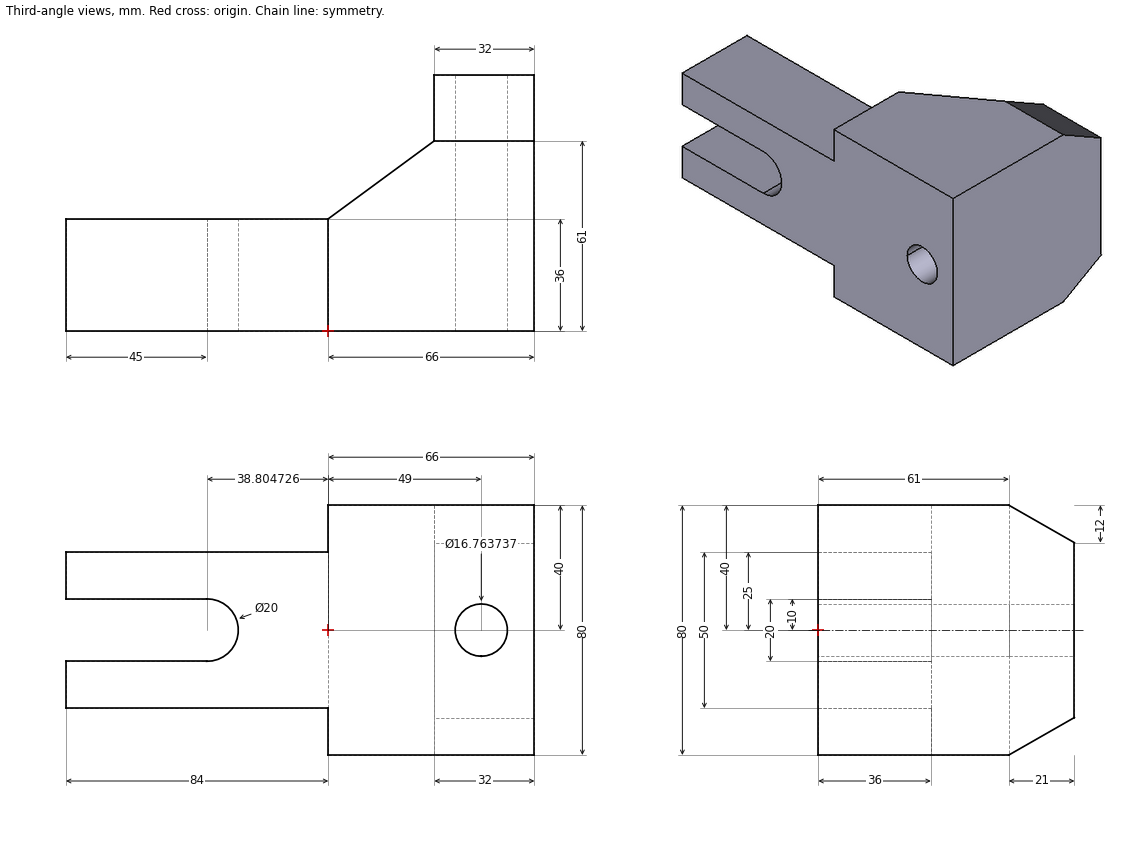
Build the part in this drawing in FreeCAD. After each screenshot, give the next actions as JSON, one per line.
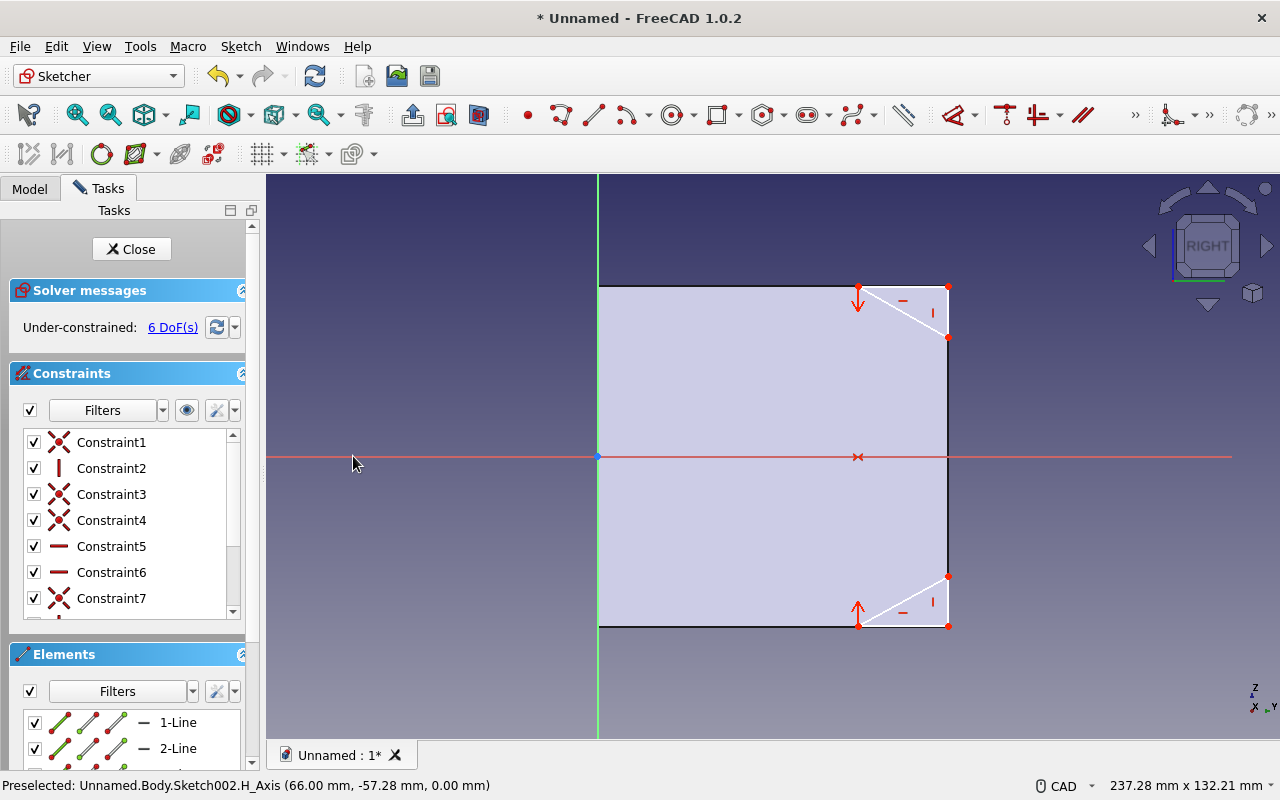
{"action": "left_click", "coordinate": [948, 338]}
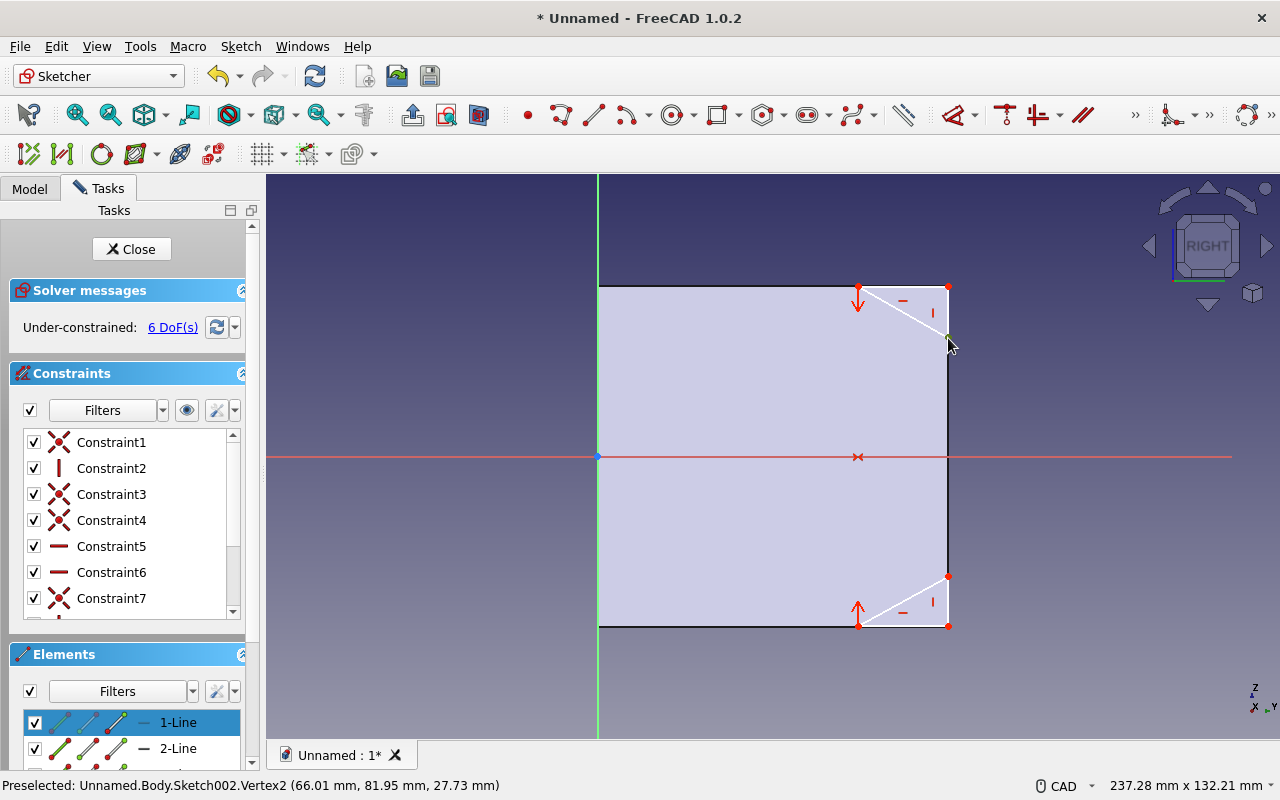
{"action": "left_click", "coordinate": [948, 577]}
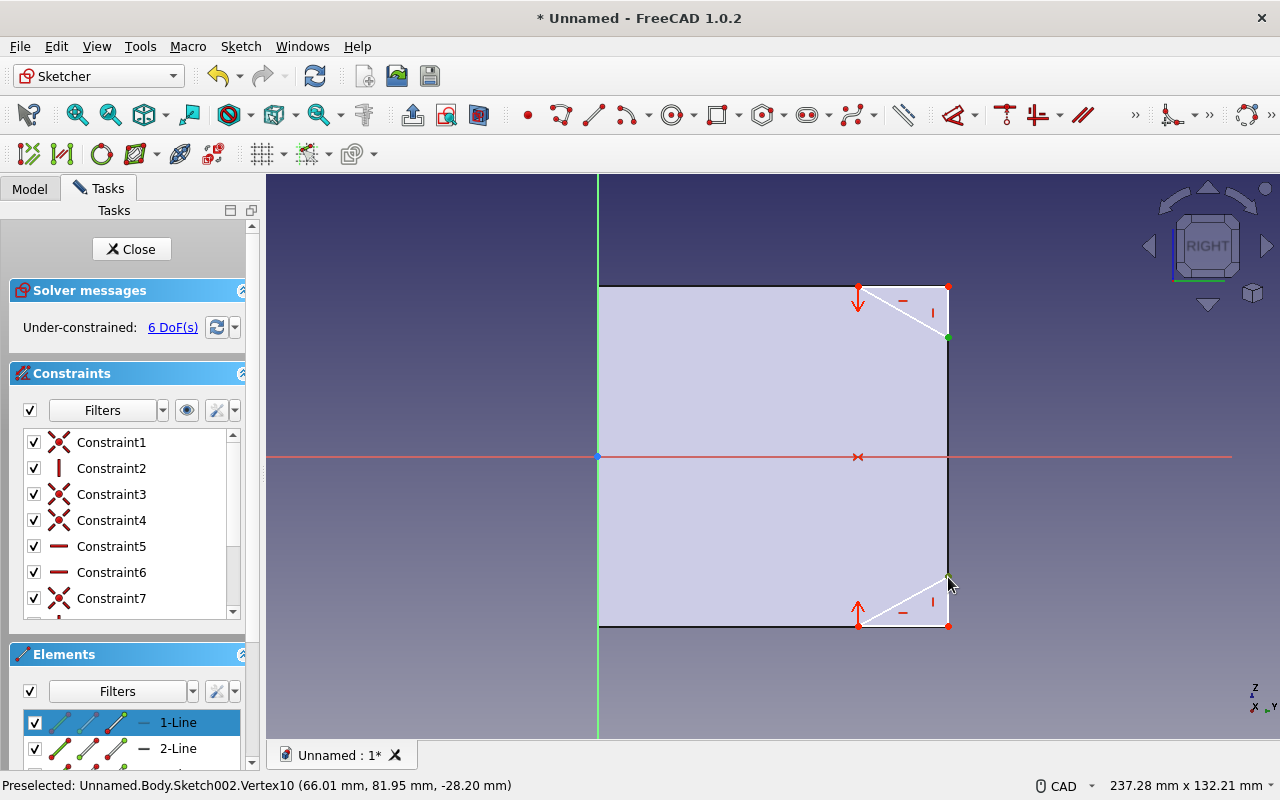
{"action": "left_click", "coordinate": [353, 456]}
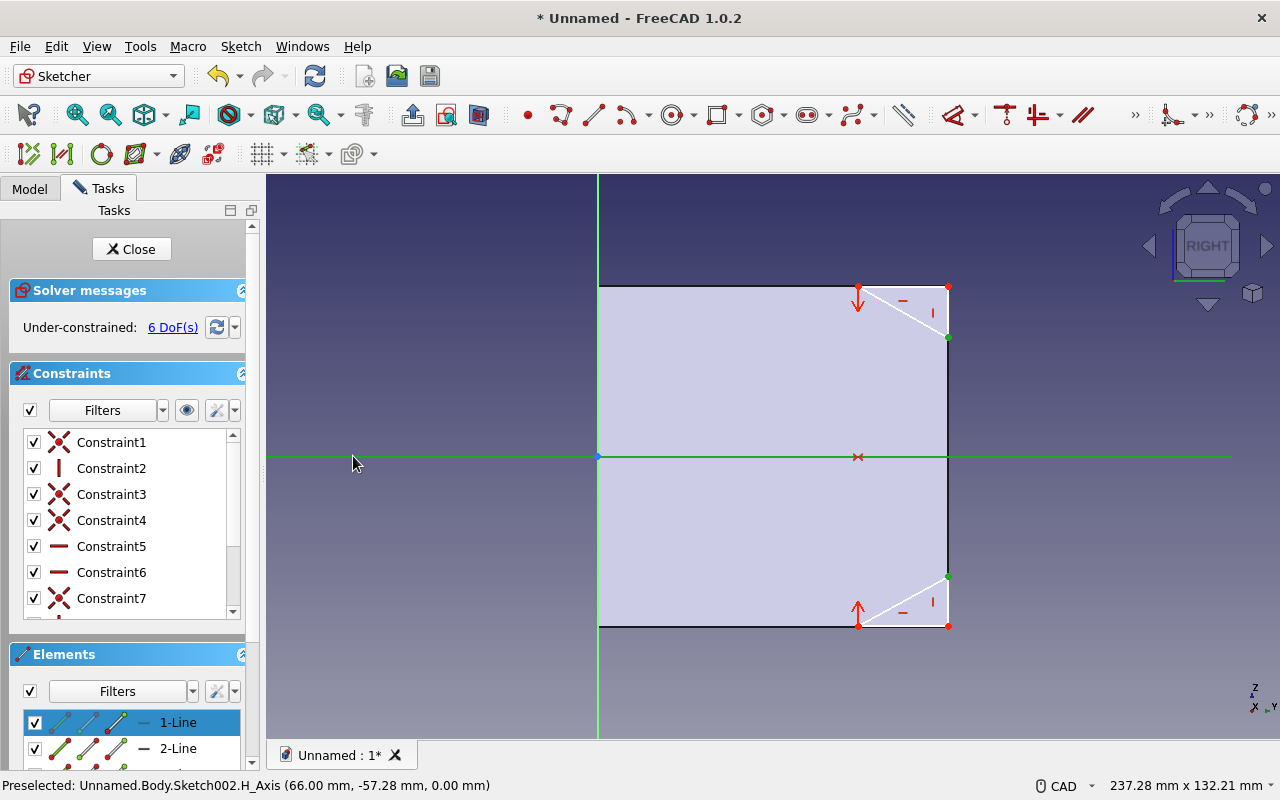
{"action": "key", "text": "s"}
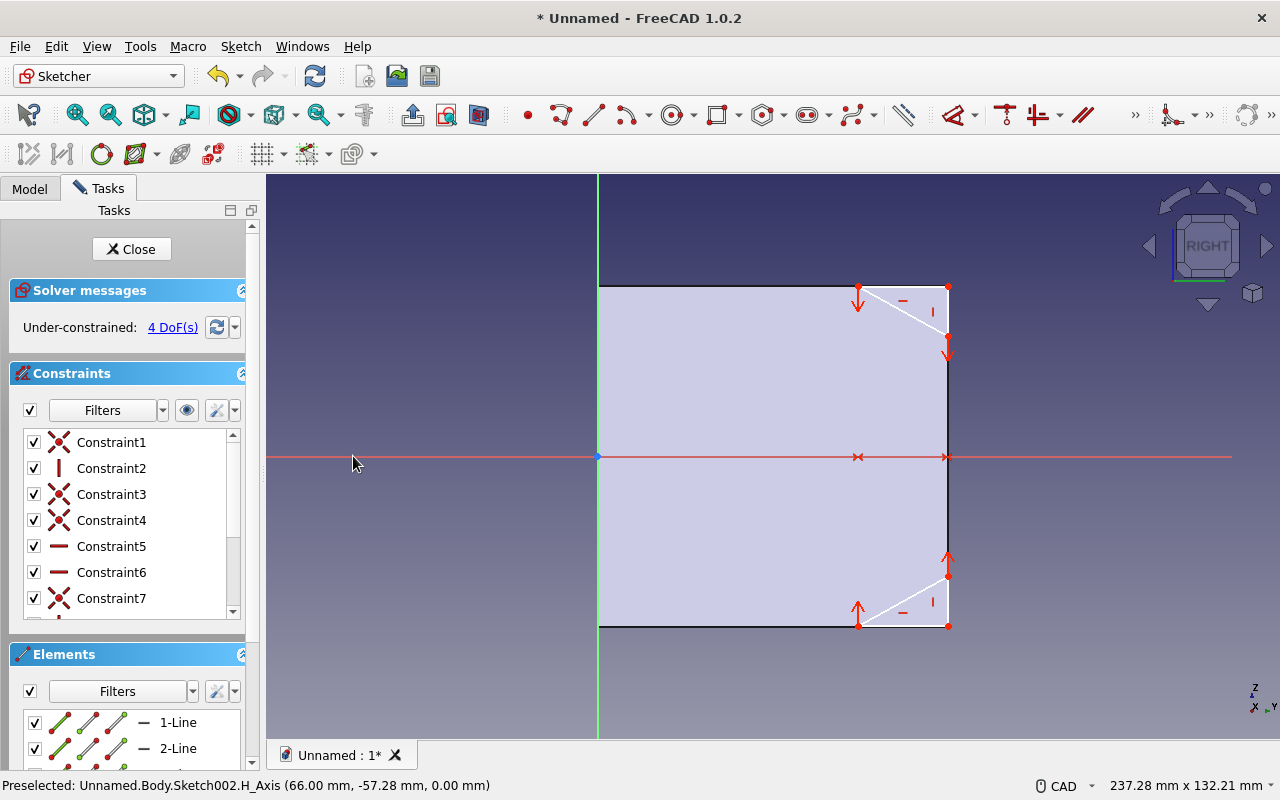
{"action": "key", "text": "d"}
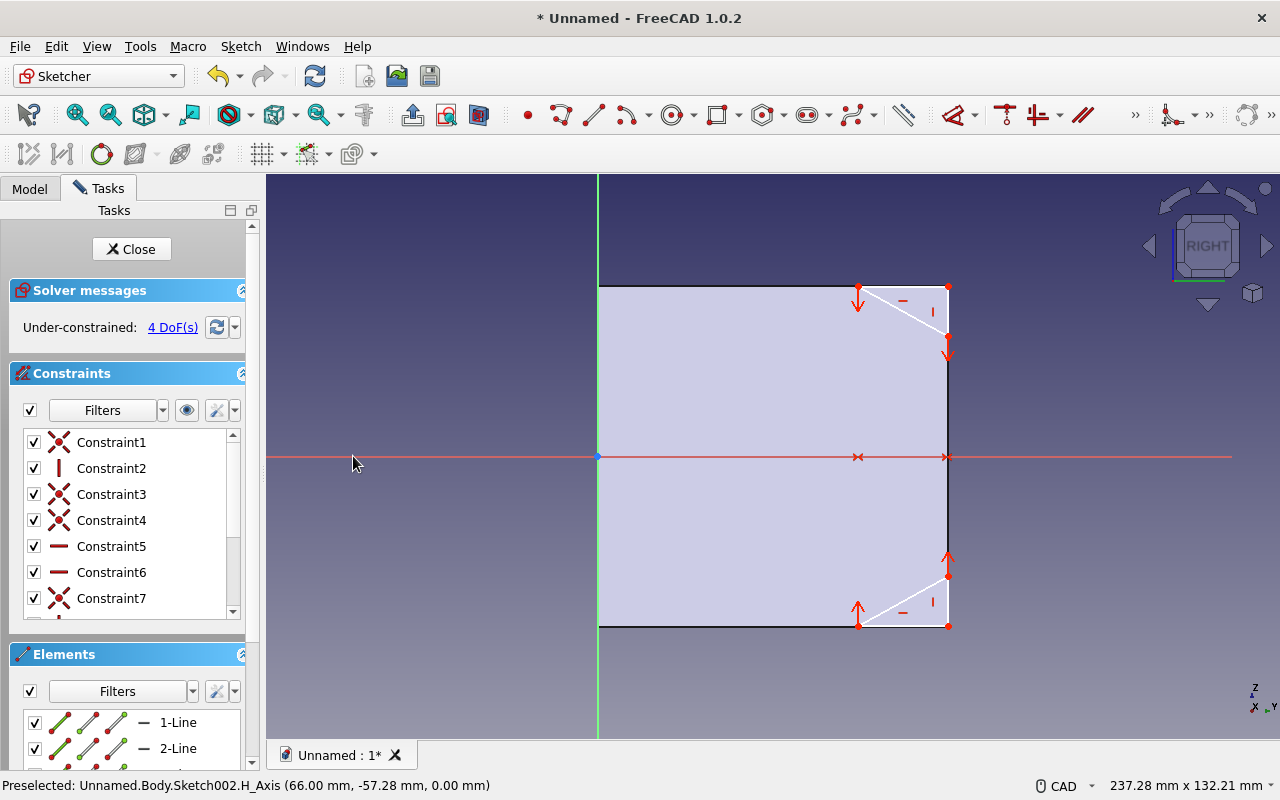
{"action": "left_click", "coordinate": [948, 321]}
{"action": "left_click", "coordinate": [982, 312]}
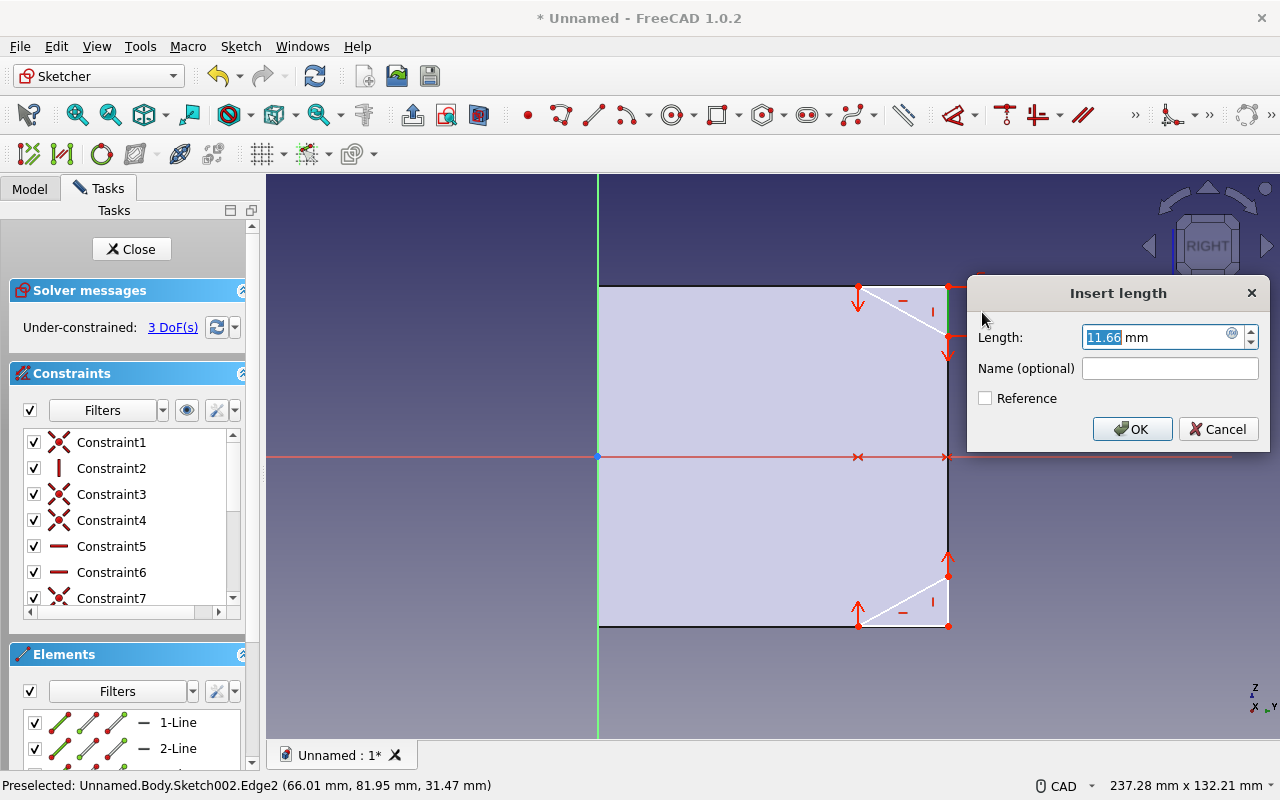
{"action": "type", "text": "12"}
{"action": "key", "text": "Return"}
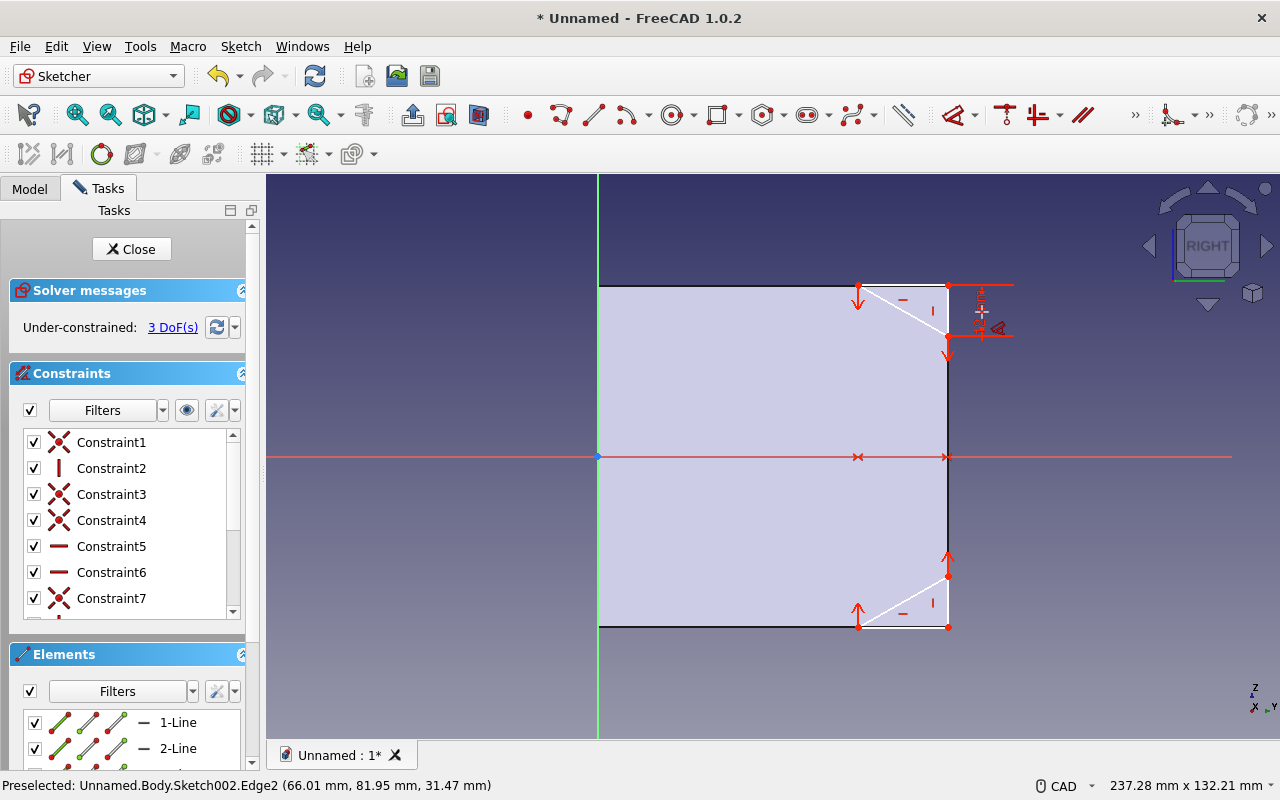
{"action": "left_click", "coordinate": [921, 285]}
{"action": "left_click", "coordinate": [903, 251]}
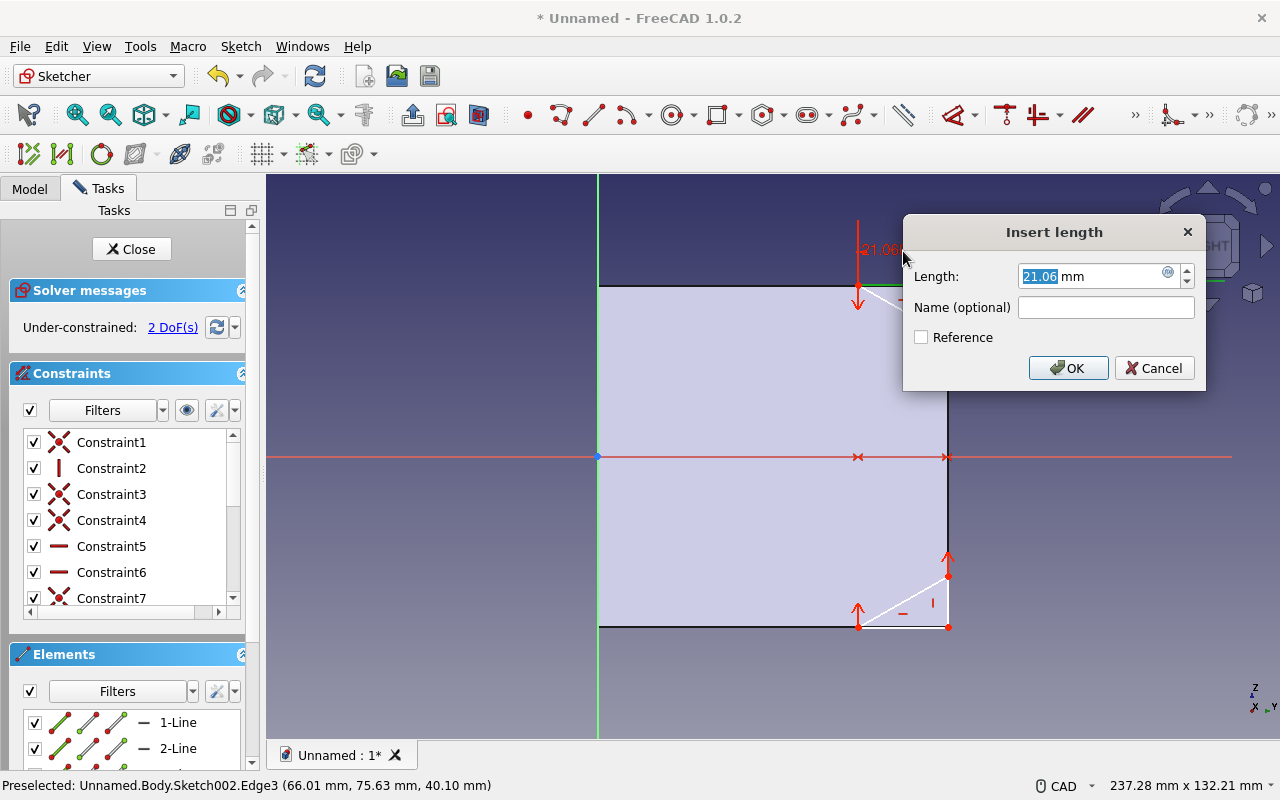
{"action": "type", "text": "21"}
{"action": "key", "text": "Return"}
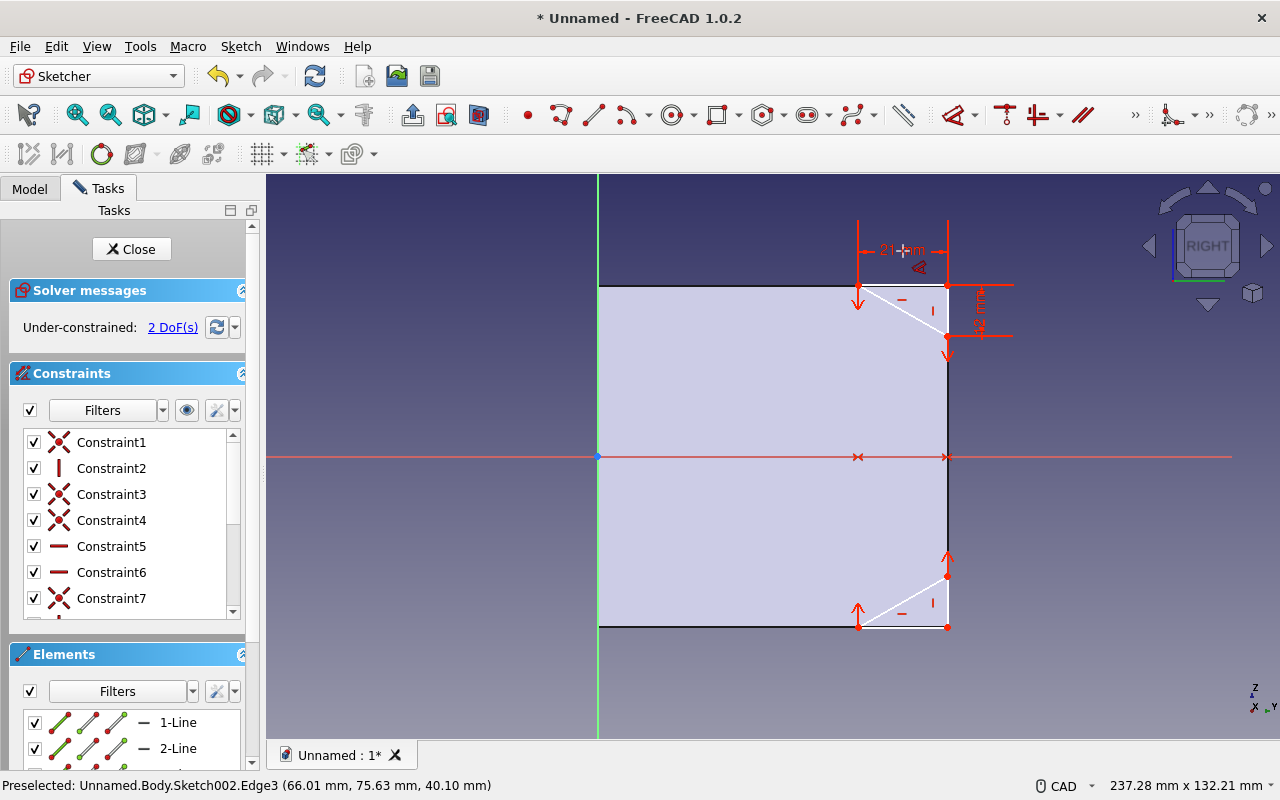
{"action": "left_click", "coordinate": [858, 285]}
{"action": "left_click", "coordinate": [728, 251]}